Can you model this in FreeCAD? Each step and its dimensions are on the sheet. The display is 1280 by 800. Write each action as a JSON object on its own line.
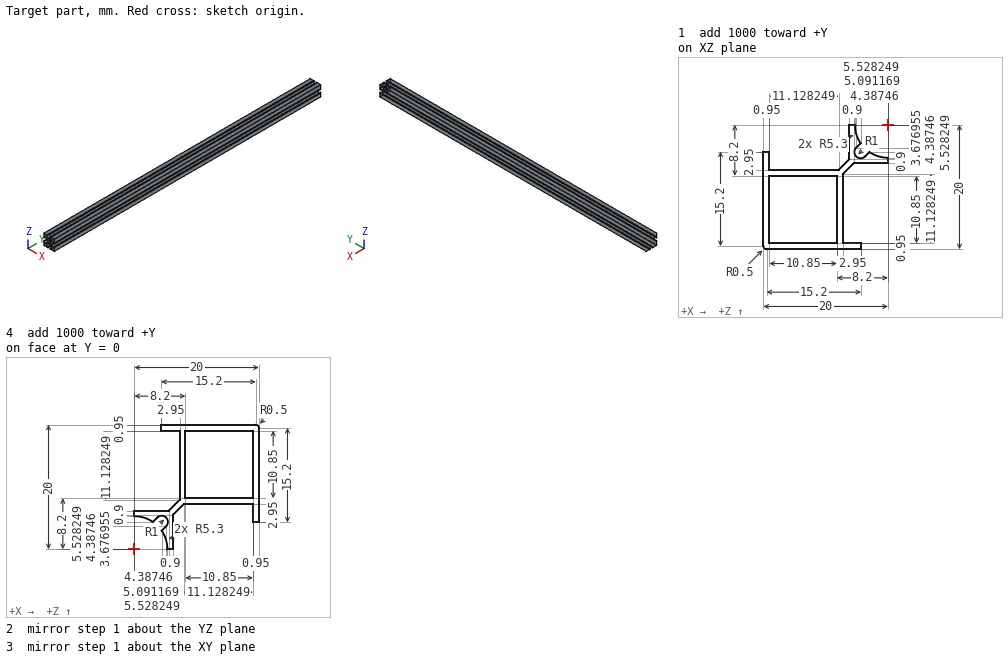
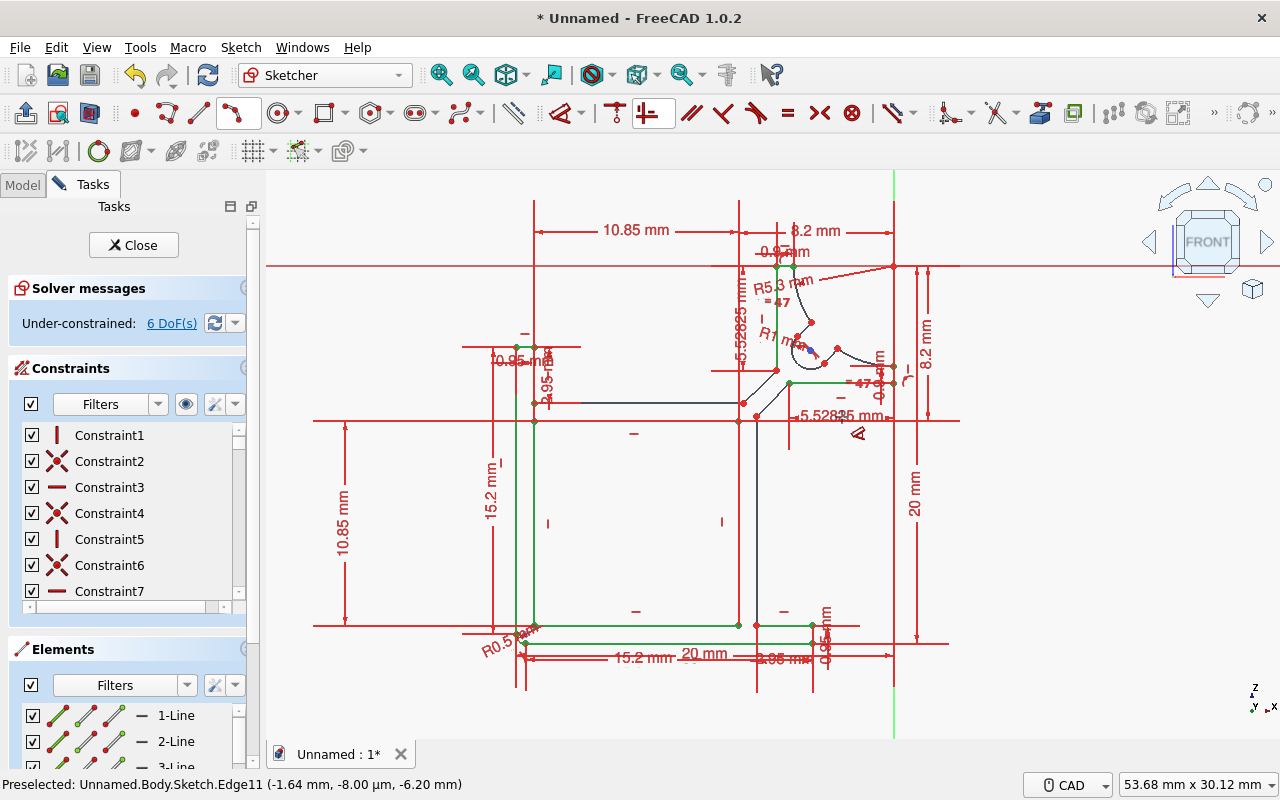
{"action": "left_click", "coordinate": [811, 323]}
{"action": "left_click", "coordinate": [853, 208]}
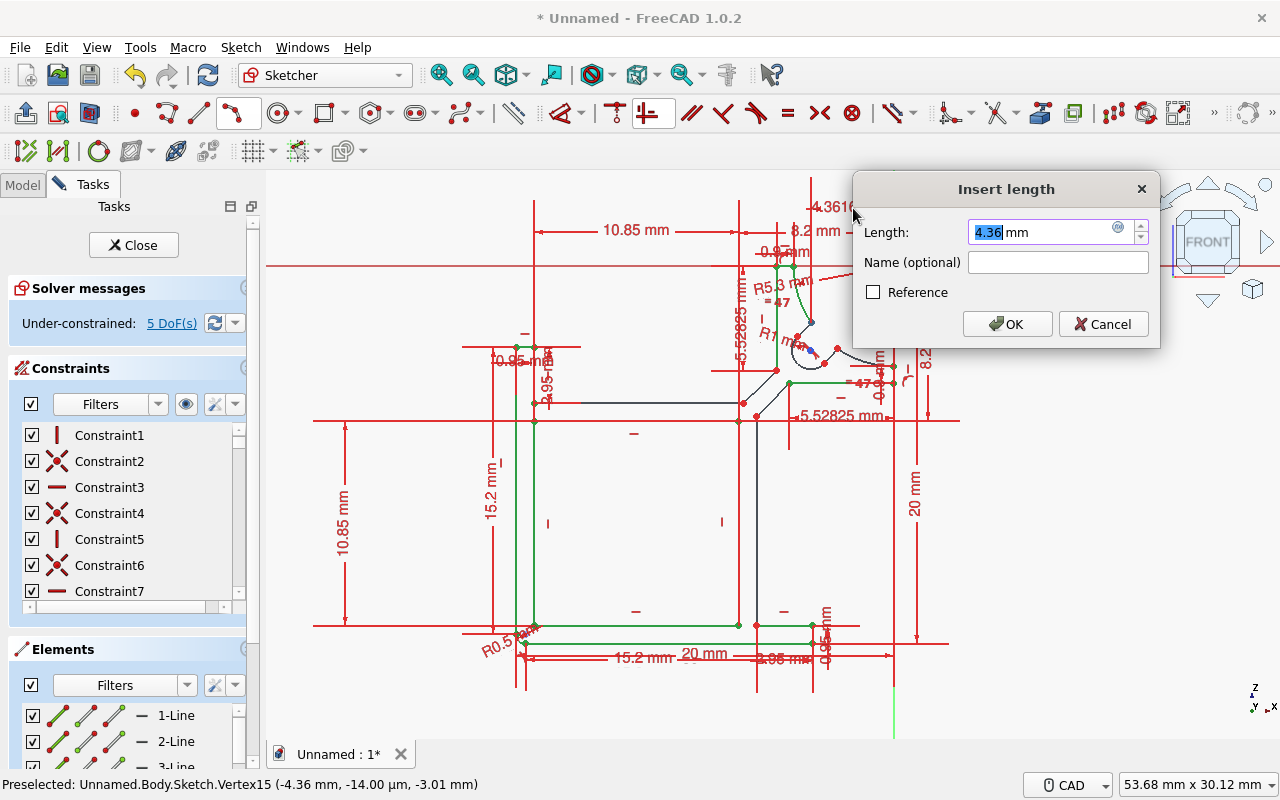
{"action": "type", "text": "4.38746"}
{"action": "key", "text": "Return"}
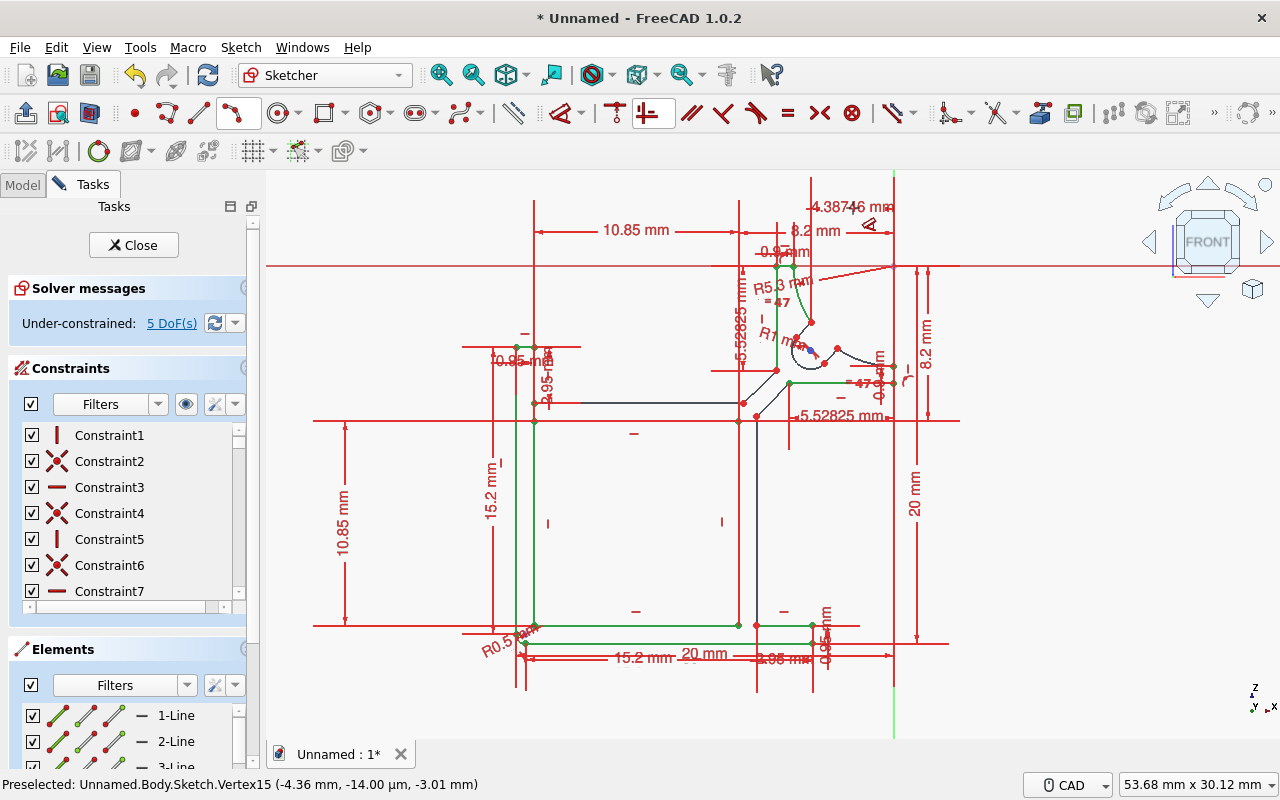
{"action": "left_click", "coordinate": [838, 349]}
{"action": "left_click", "coordinate": [928, 308]}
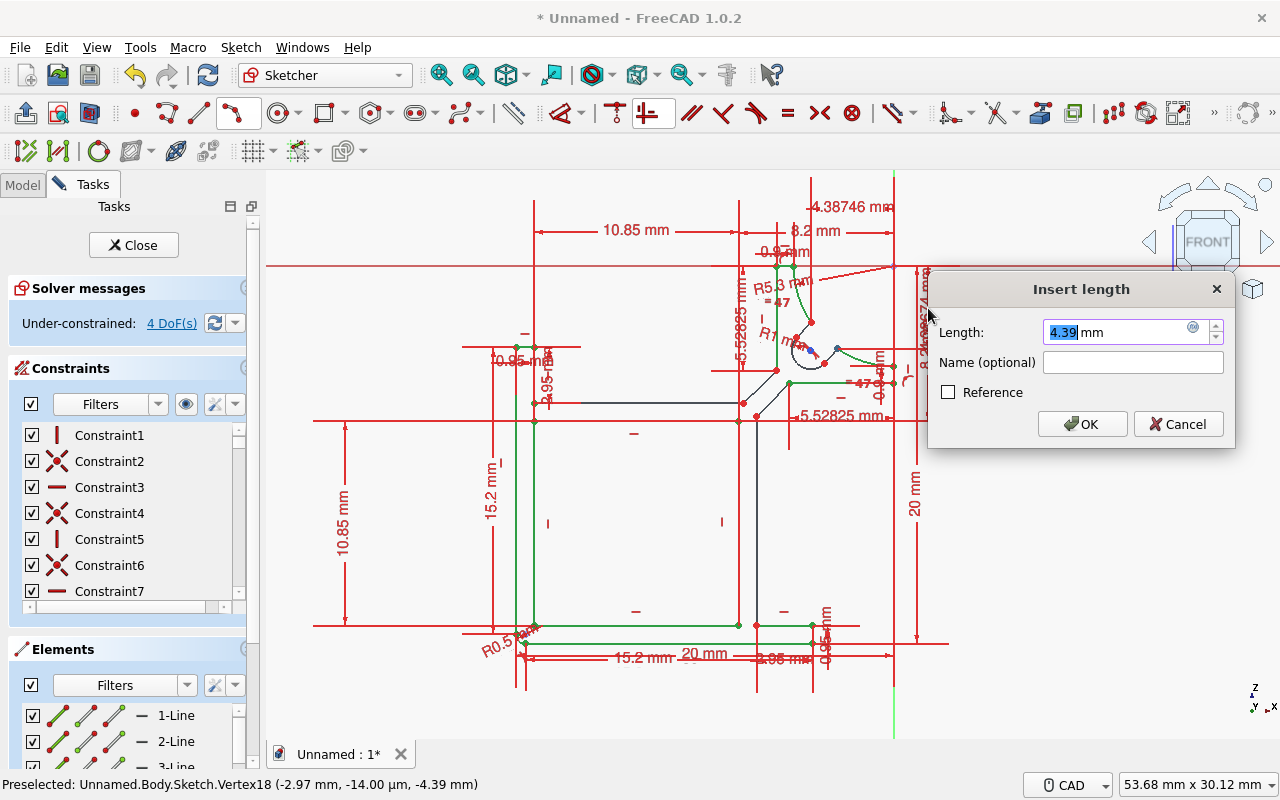
{"action": "type", "text": "4.38746"}
{"action": "key", "text": "Return"}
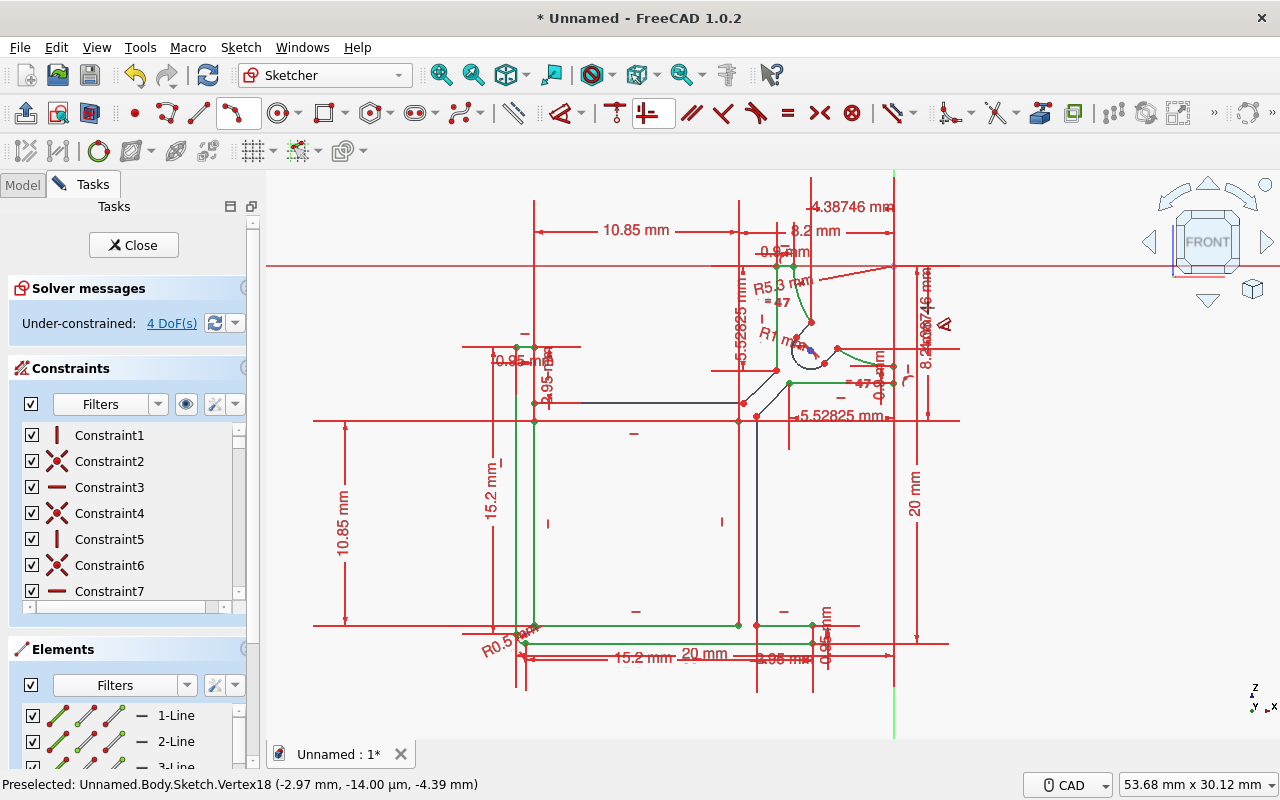
{"action": "left_click", "coordinate": [597, 403]}
{"action": "left_click", "coordinate": [639, 369]}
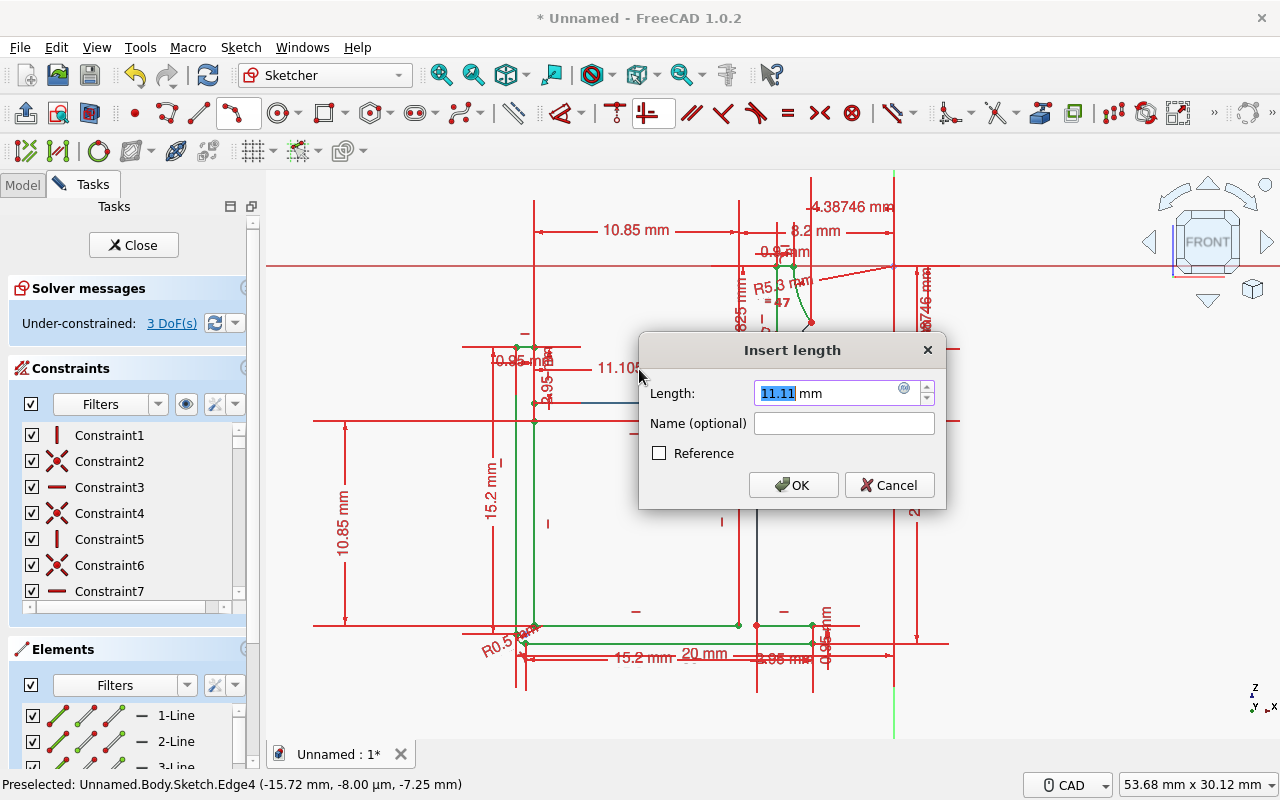
{"action": "type", "text": "11.128249"}
{"action": "key", "text": "Return"}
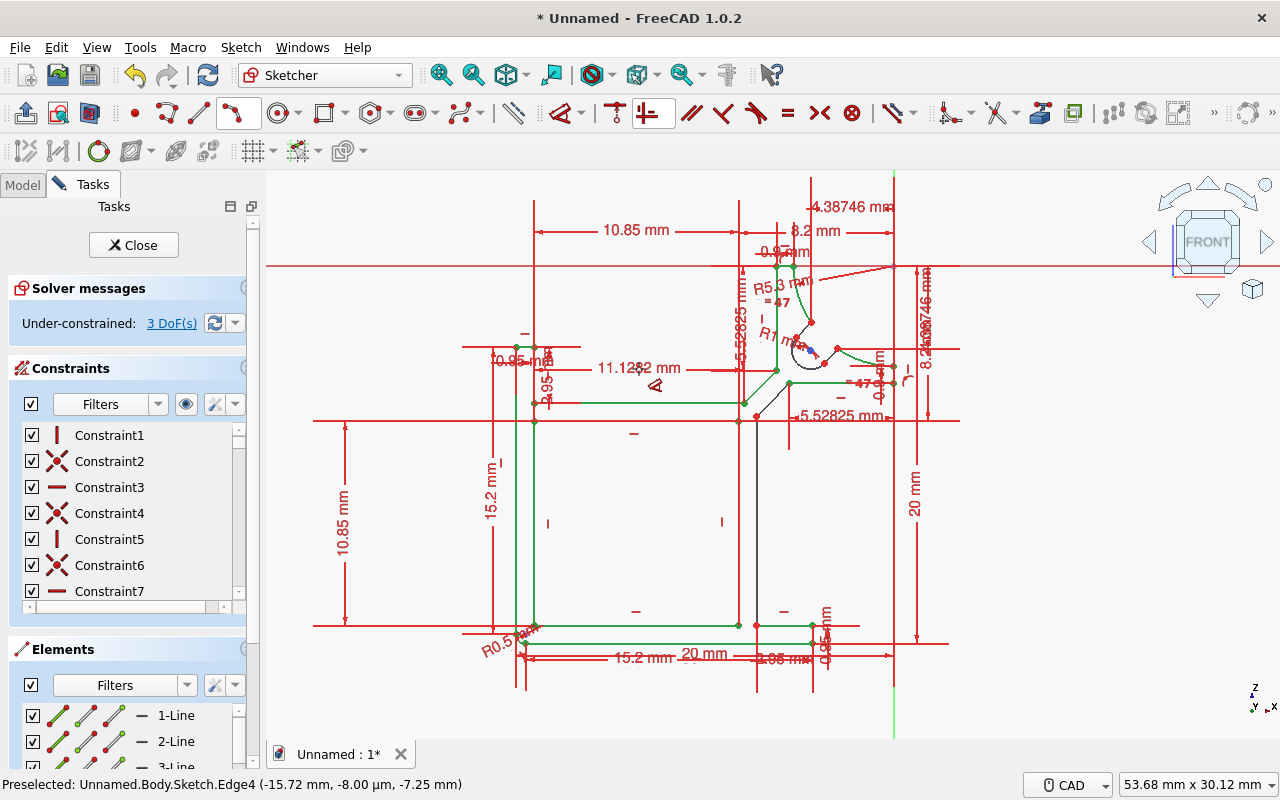
{"action": "left_click", "coordinate": [757, 479]}
{"action": "left_click", "coordinate": [791, 521]}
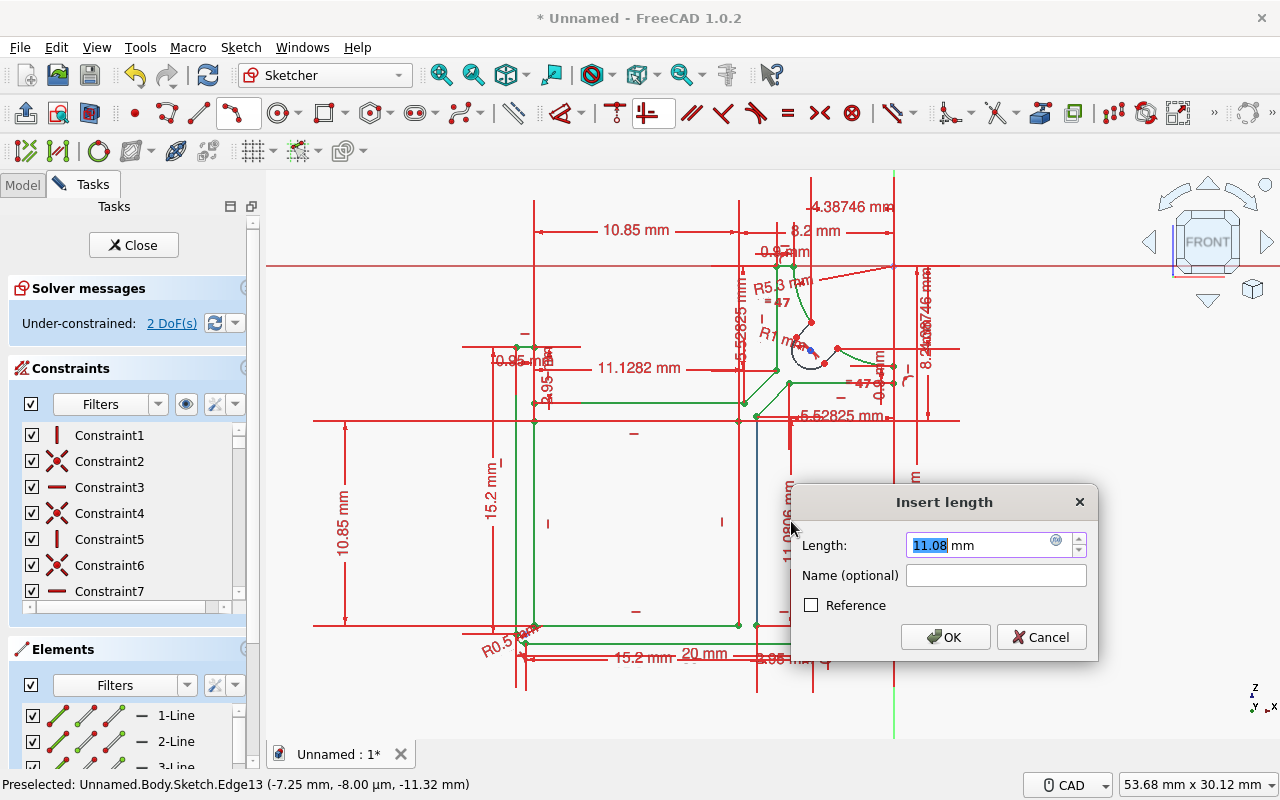
{"action": "type", "text": "11.128249"}
{"action": "key", "text": "Return"}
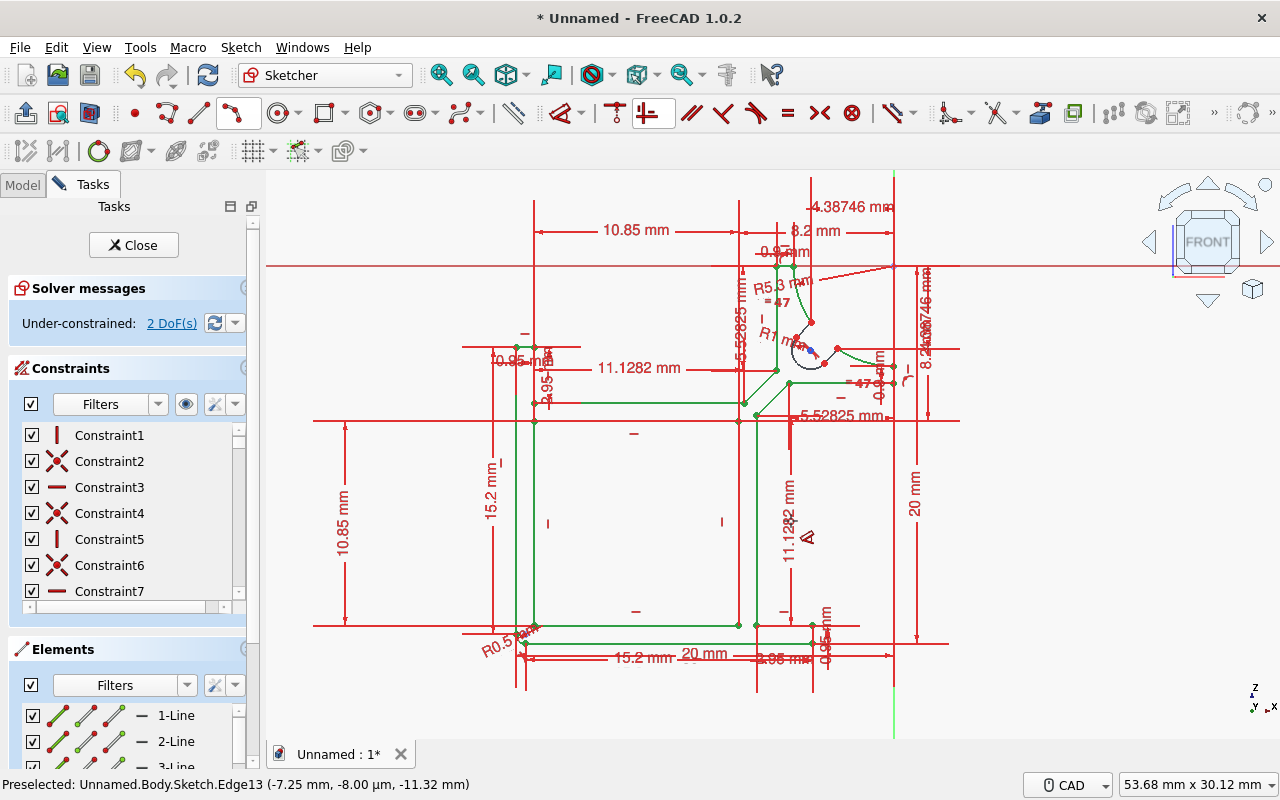
{"action": "left_click", "coordinate": [797, 338]}
{"action": "left_click", "coordinate": [845, 444]}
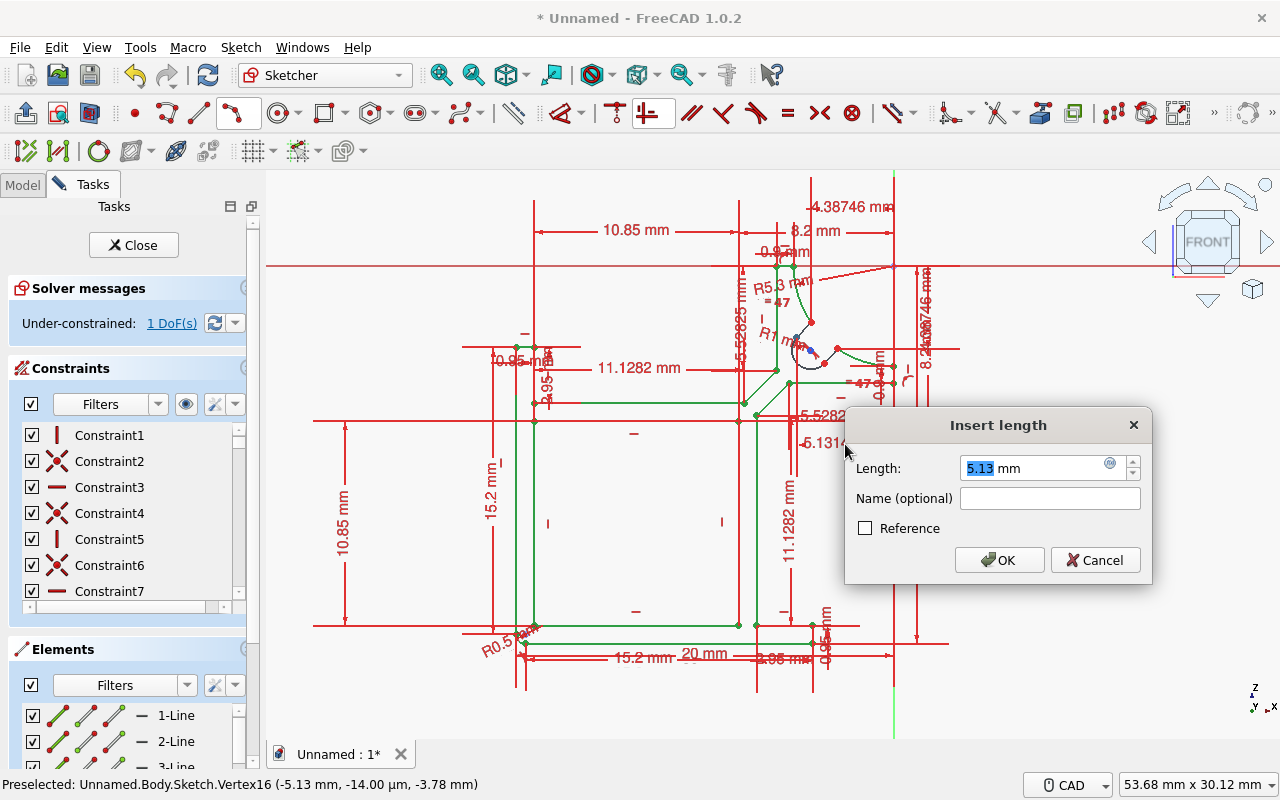
{"action": "type", "text": "5.091169"}
{"action": "key", "text": "Return"}